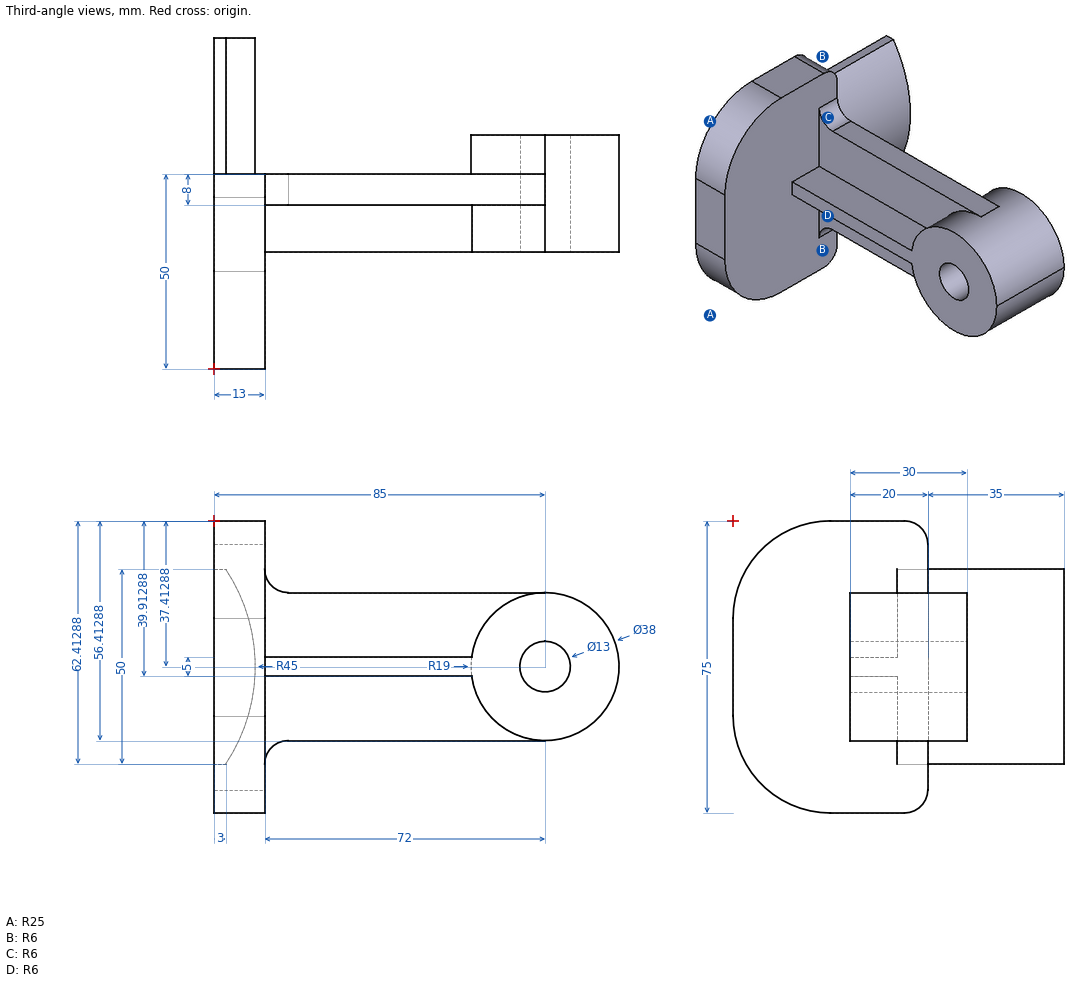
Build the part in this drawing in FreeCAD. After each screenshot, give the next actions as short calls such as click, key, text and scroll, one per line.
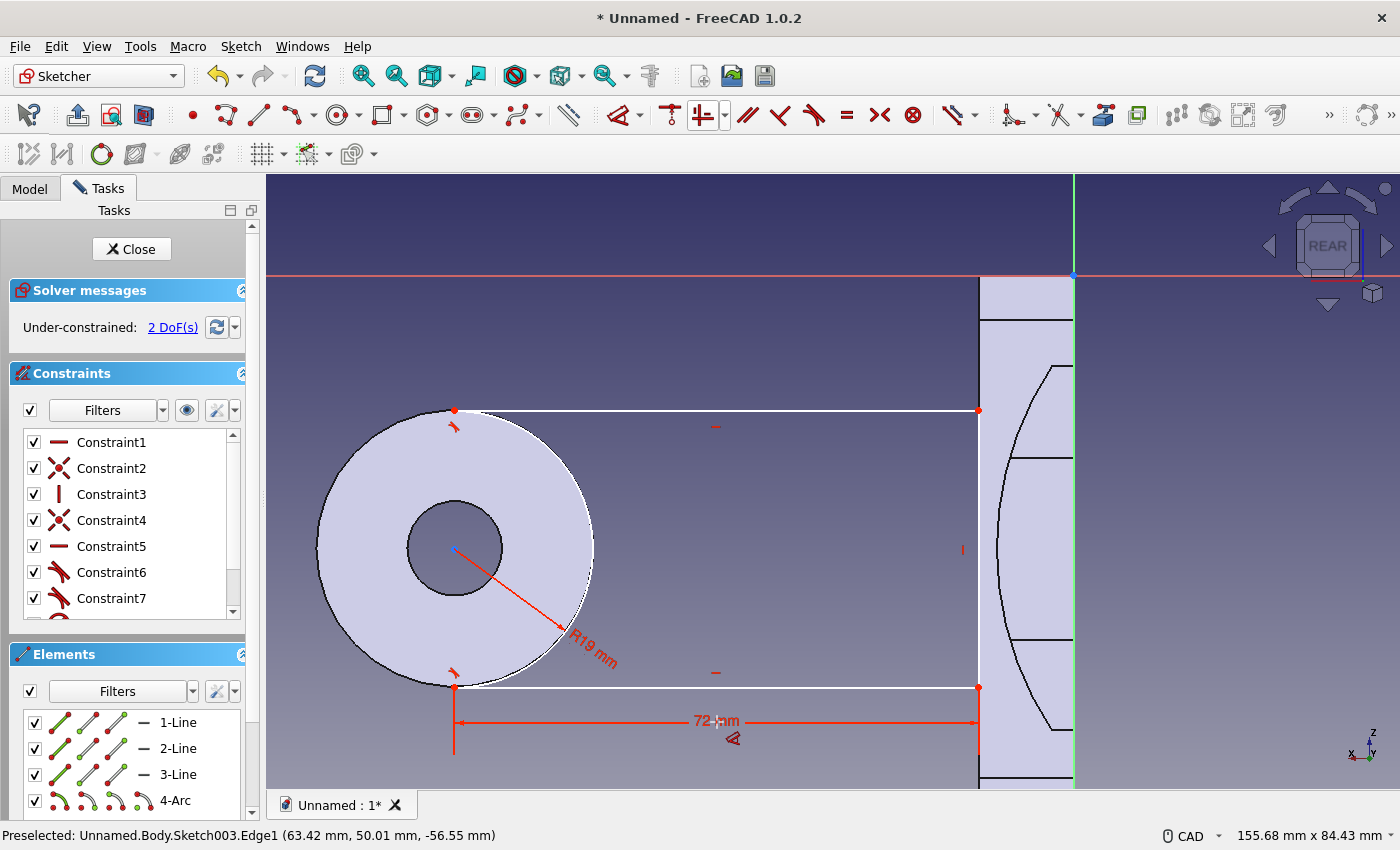
click(455, 688)
click(622, 722)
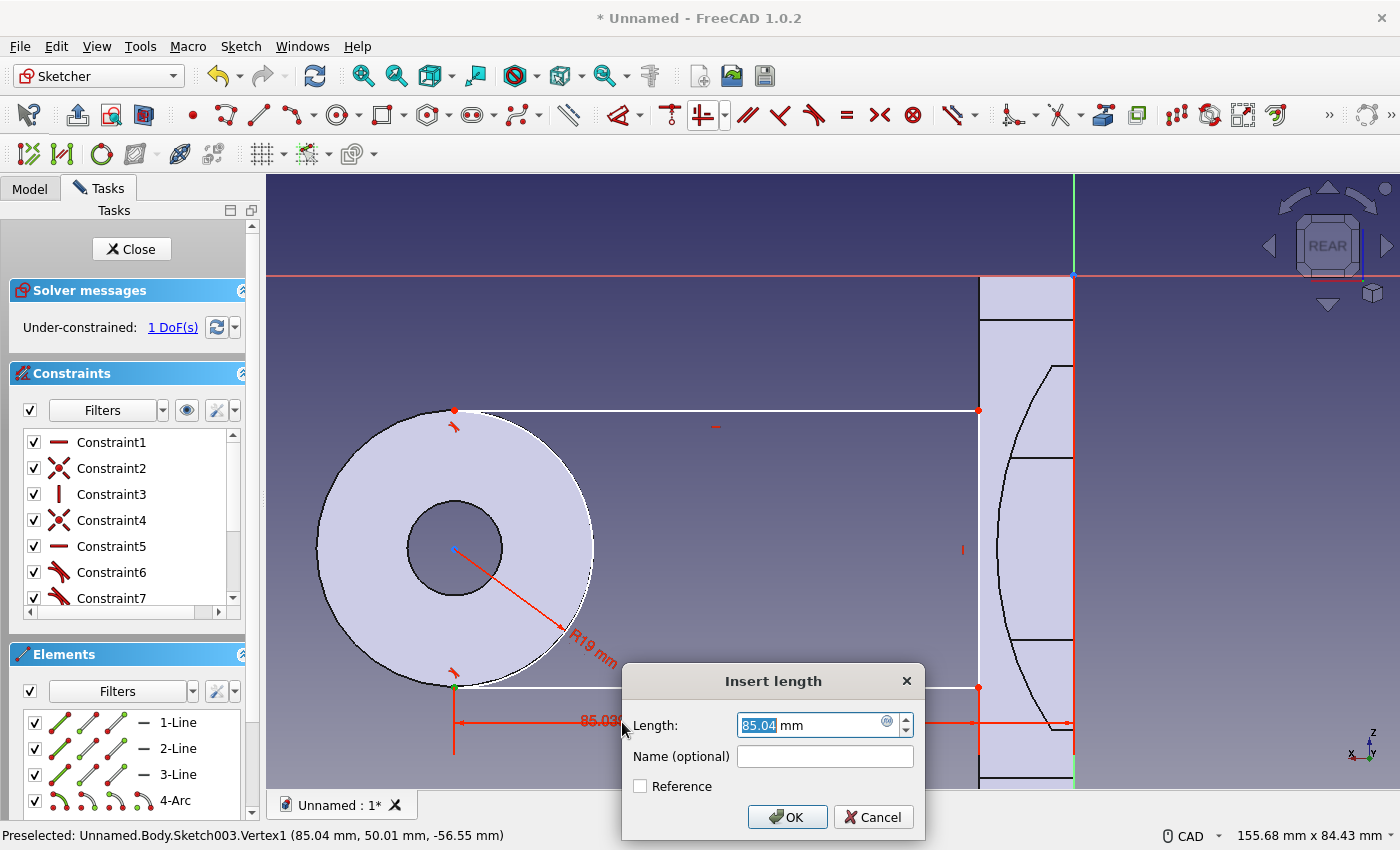
text(85)
key(Return)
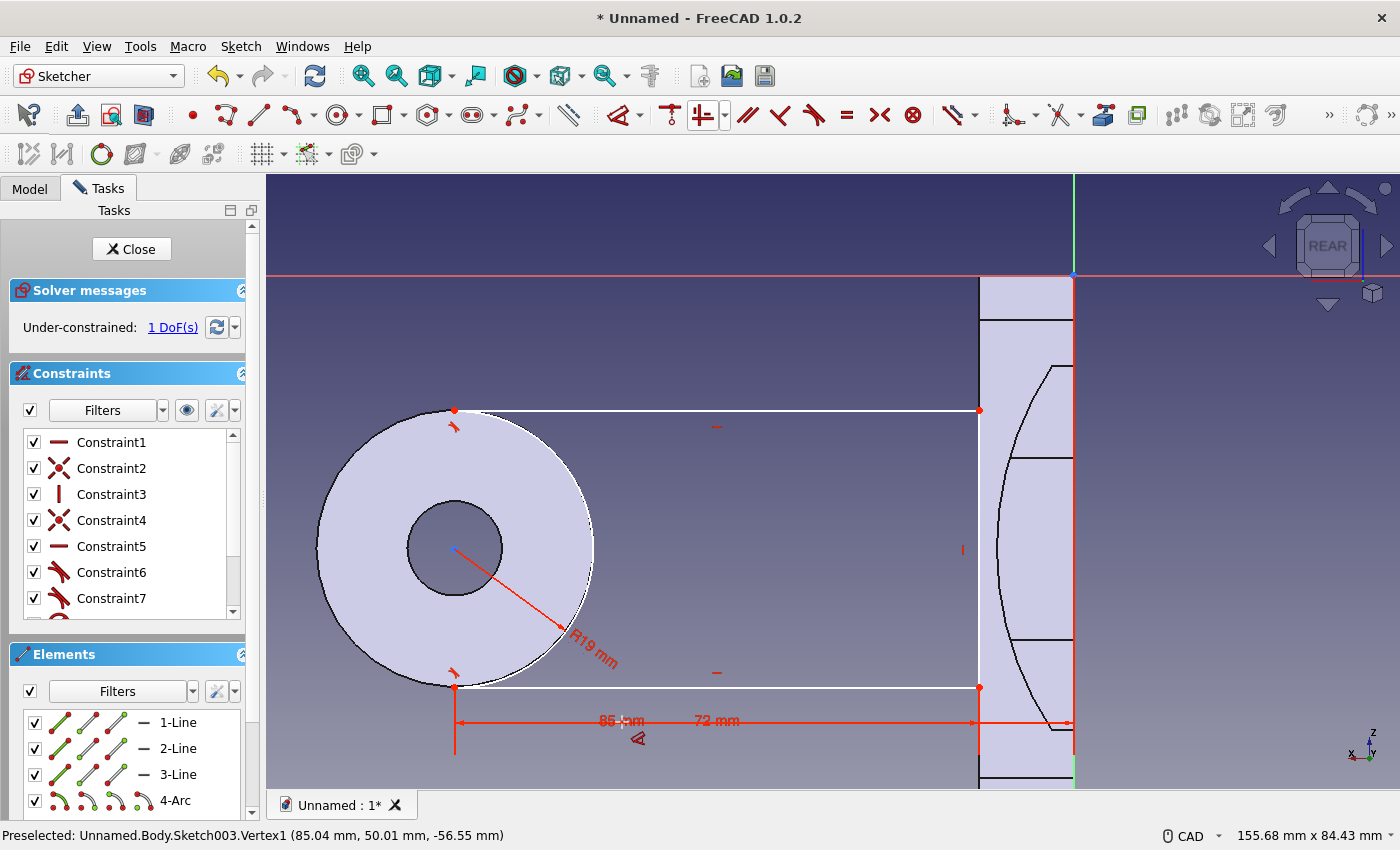
click(455, 688)
click(1108, 482)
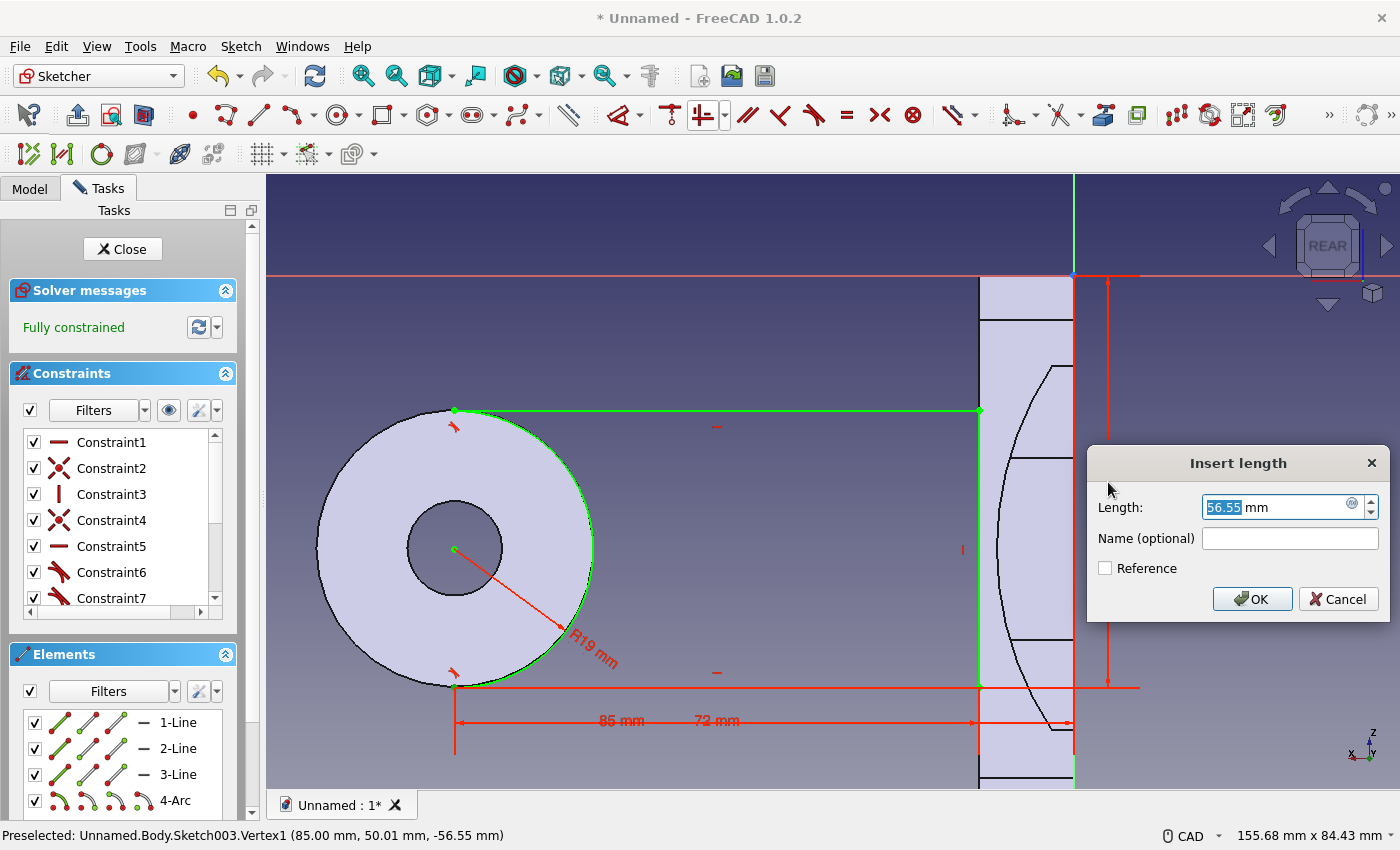
text(56.41288)
key(Return)
key(Escape)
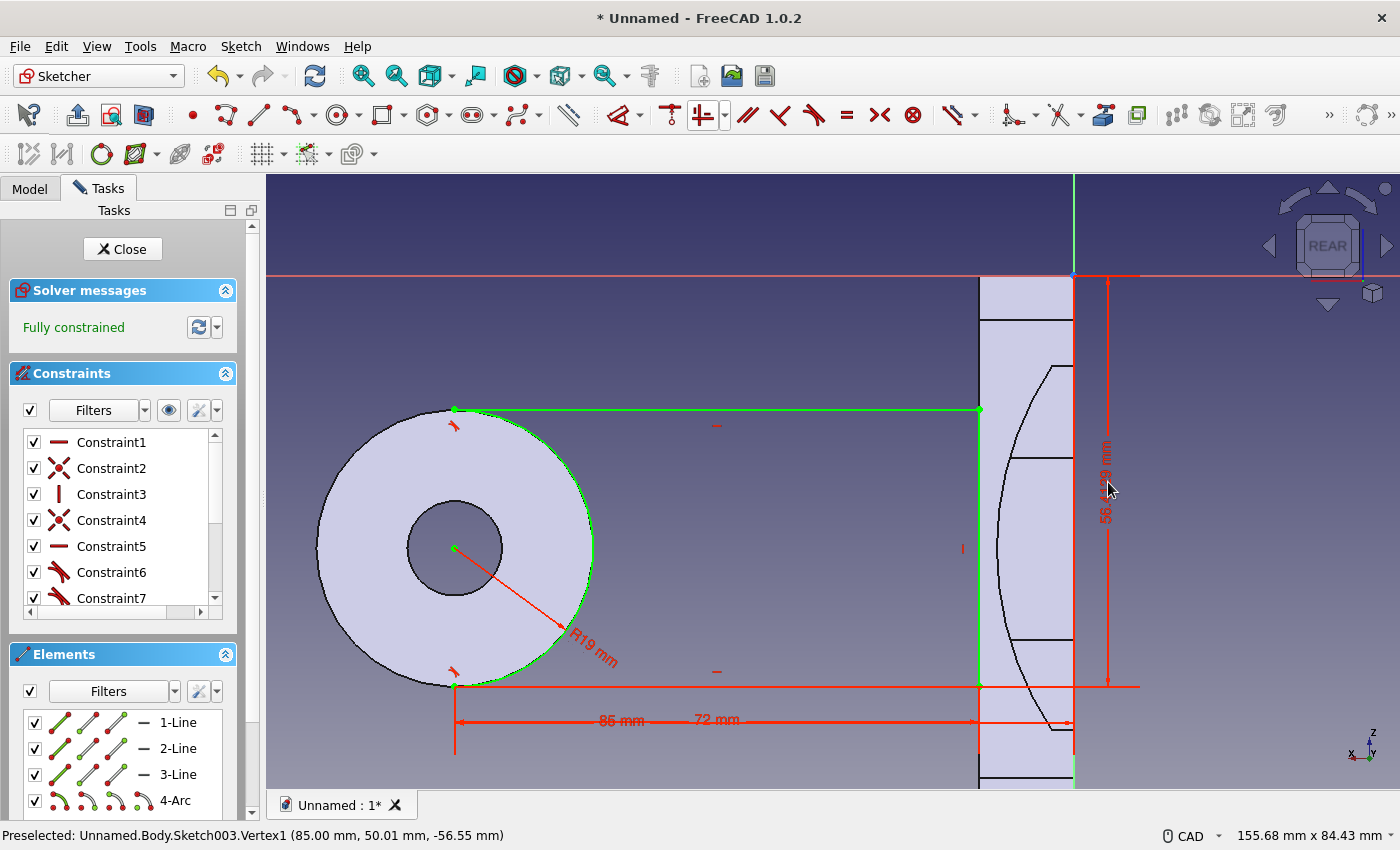
click(123, 249)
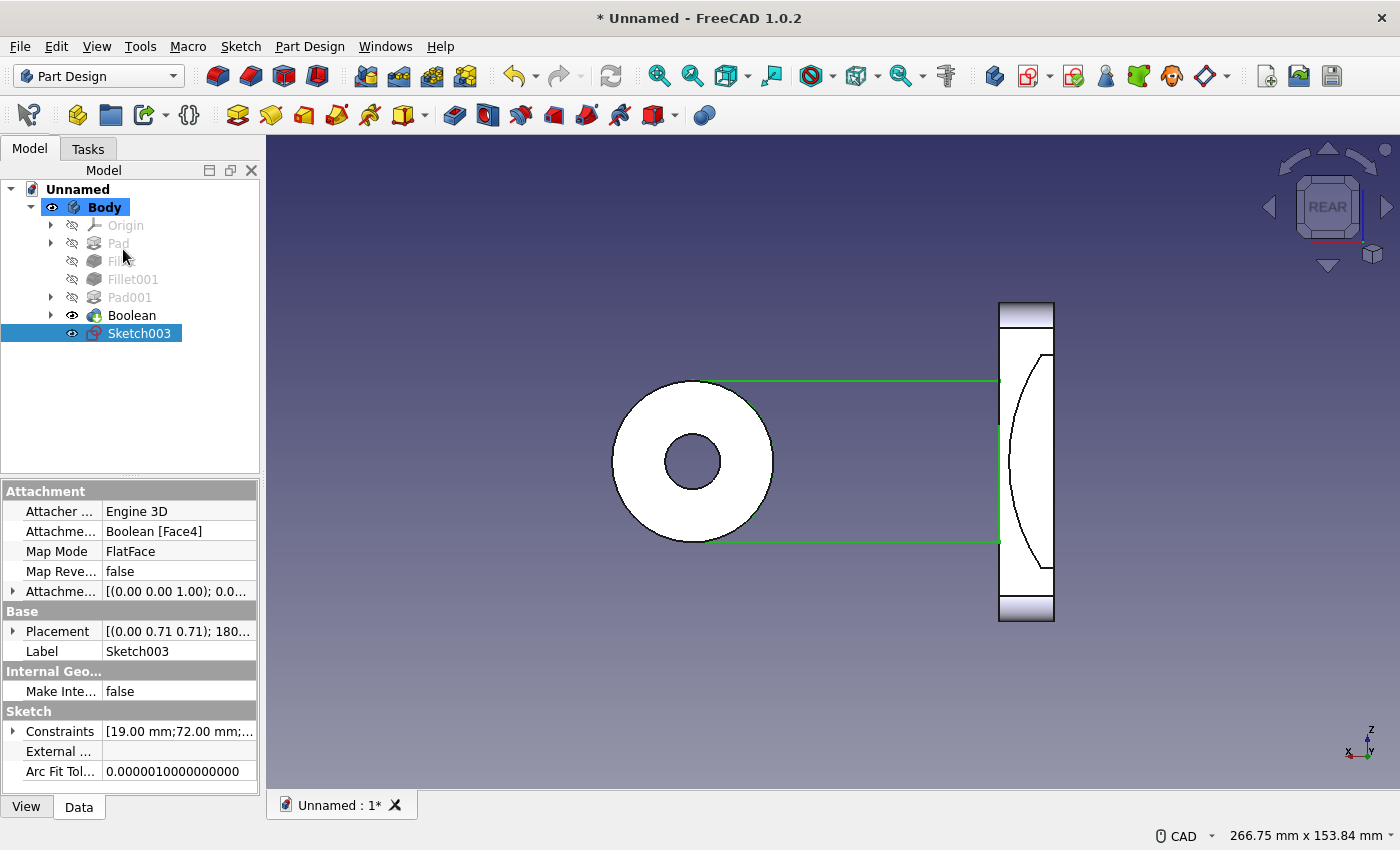
click(238, 116)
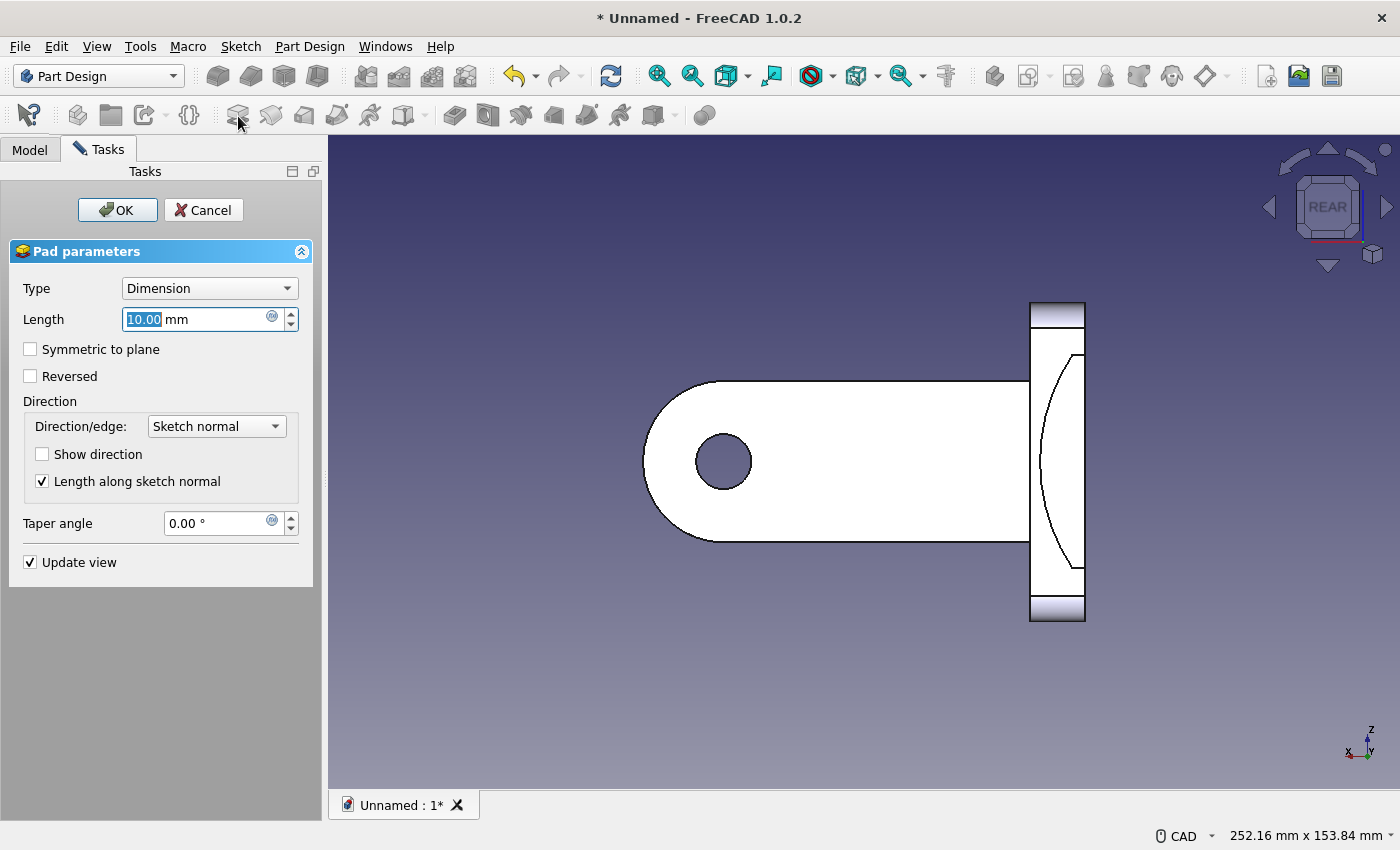
text(8)
key(Tab)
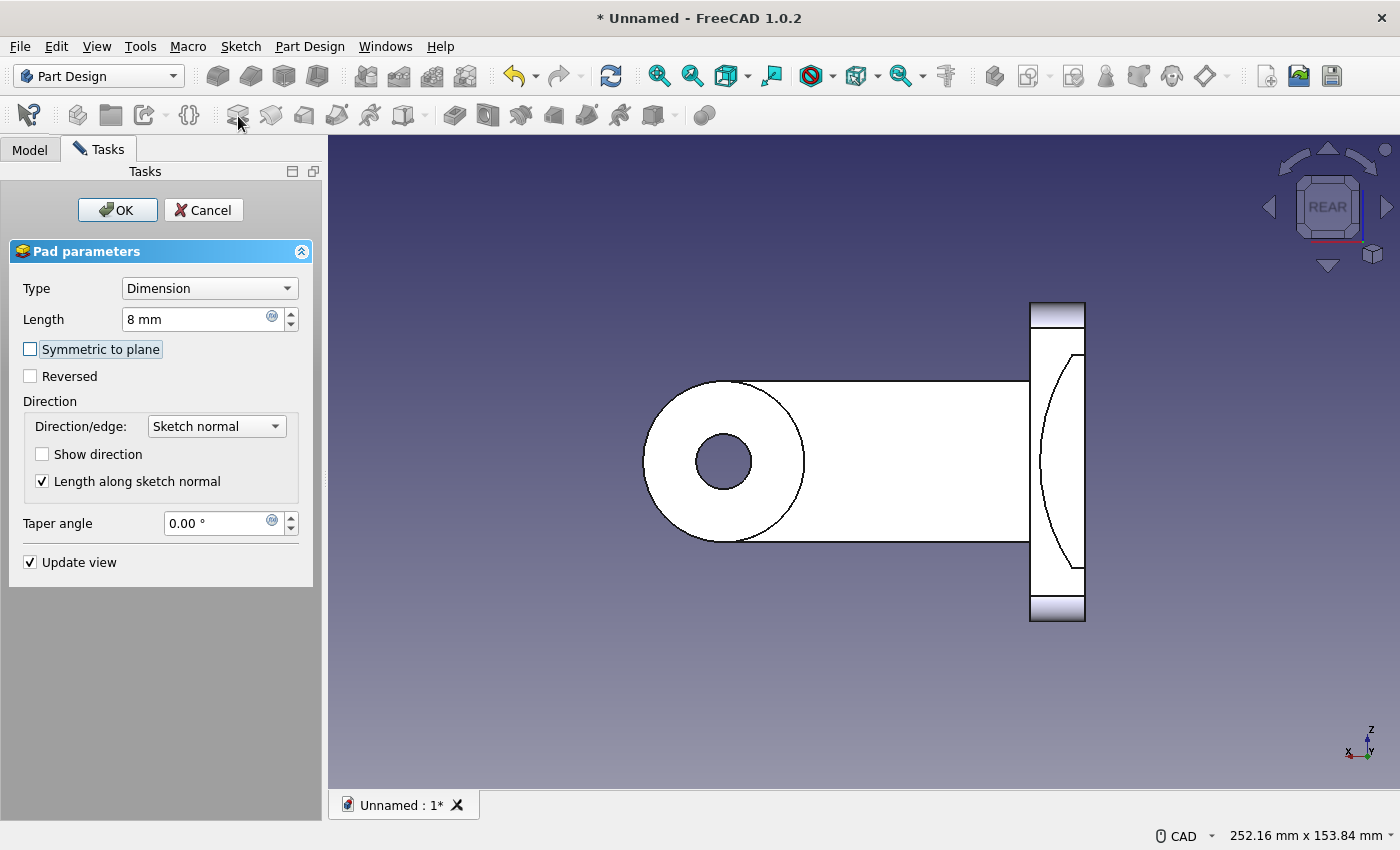
click(31, 376)